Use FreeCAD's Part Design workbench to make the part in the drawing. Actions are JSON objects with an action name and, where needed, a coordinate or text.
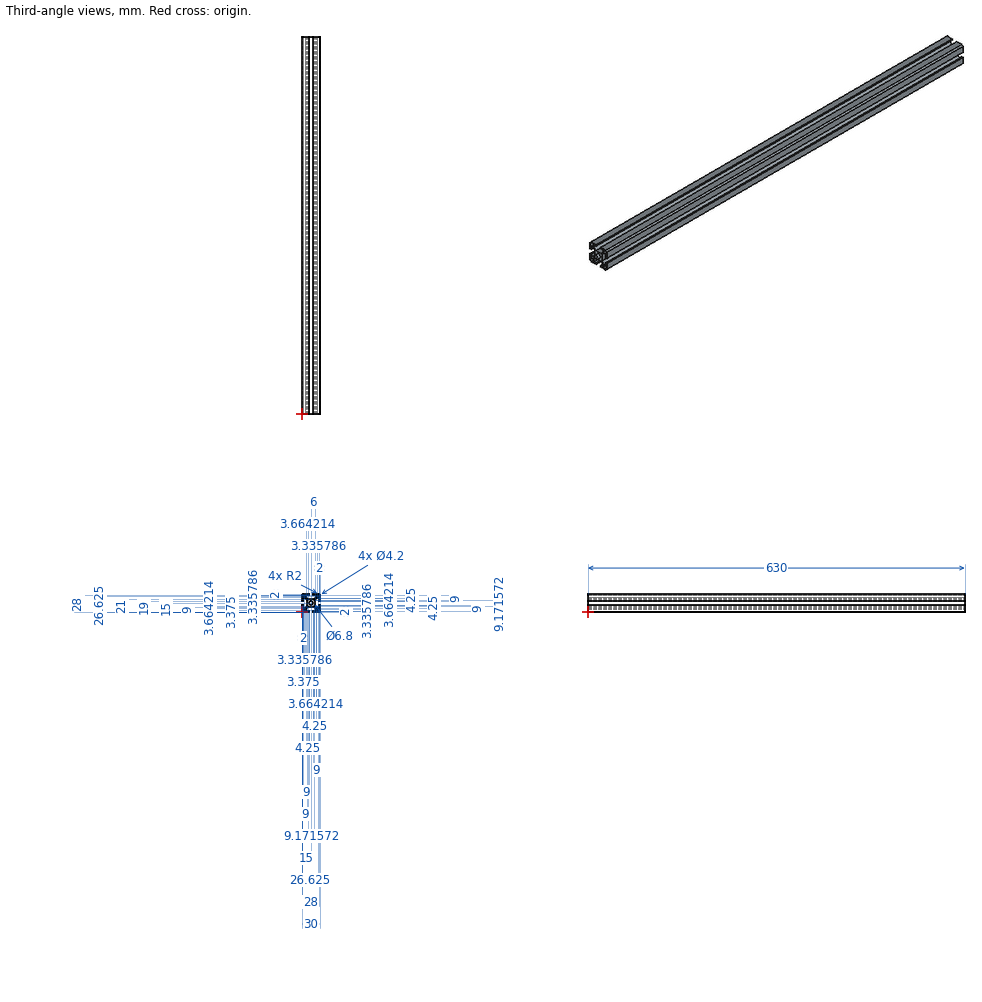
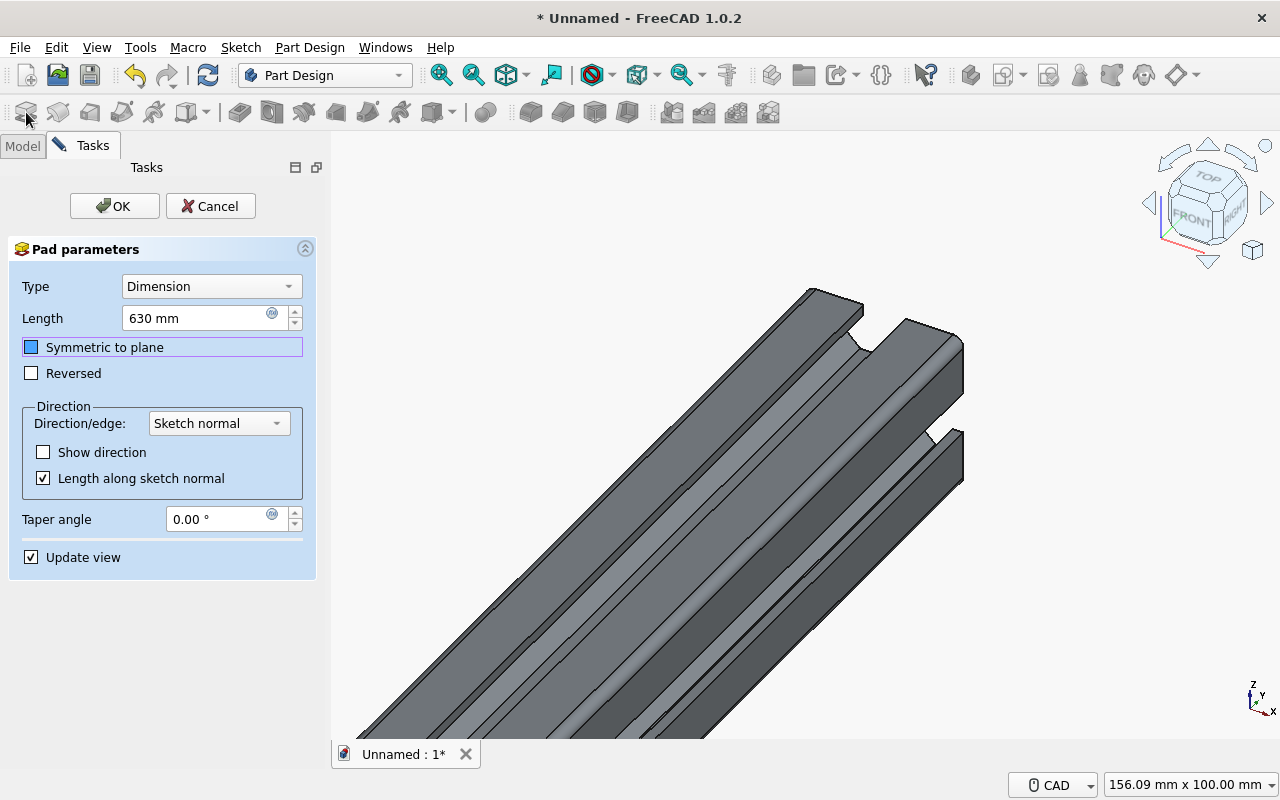
{"action": "left_click", "coordinate": [30, 373]}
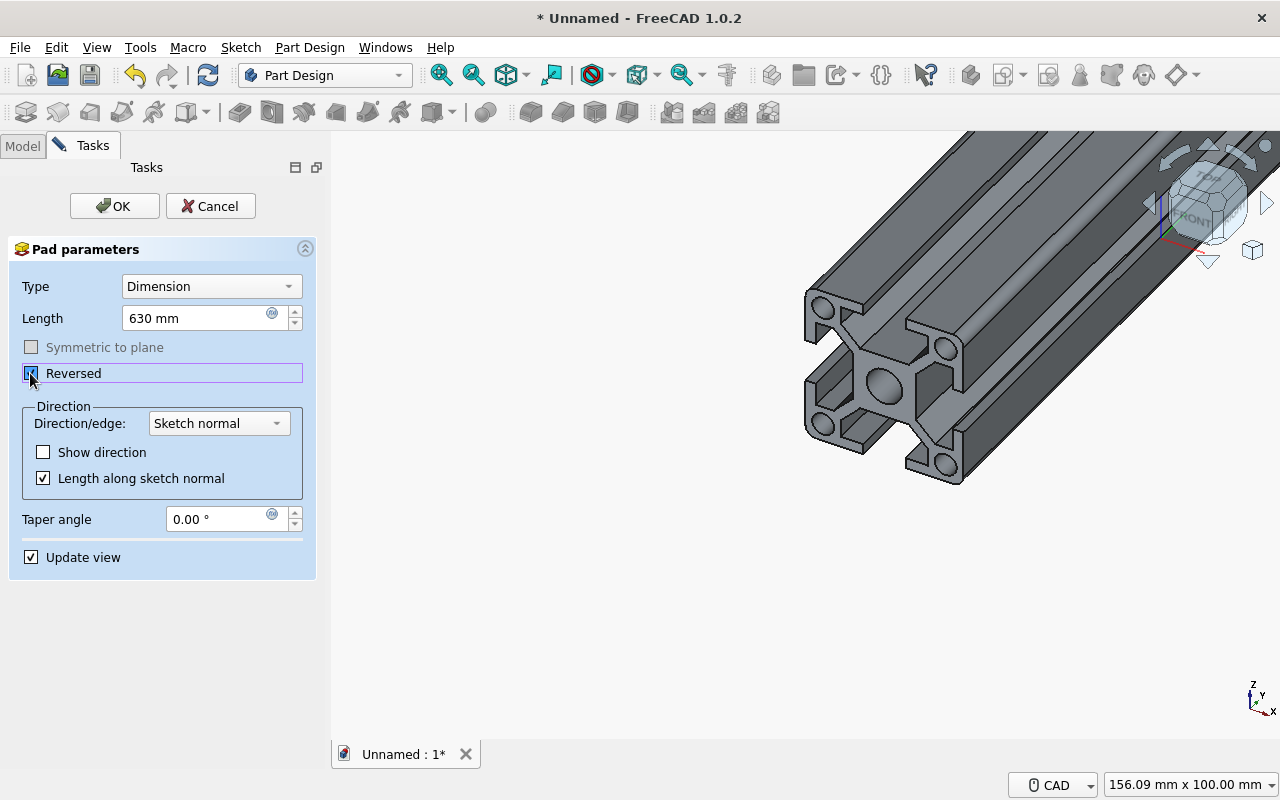
{"action": "left_click", "coordinate": [115, 206]}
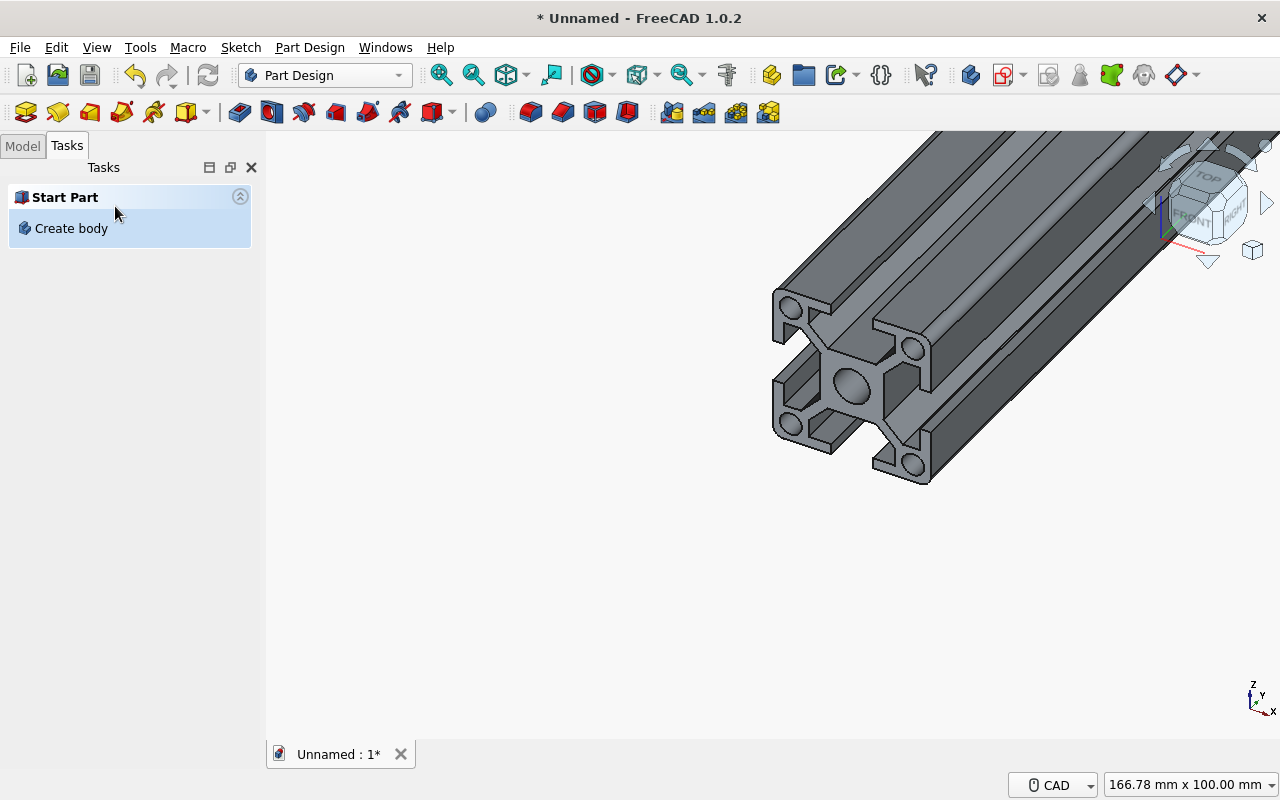
{"action": "key", "text": "0"}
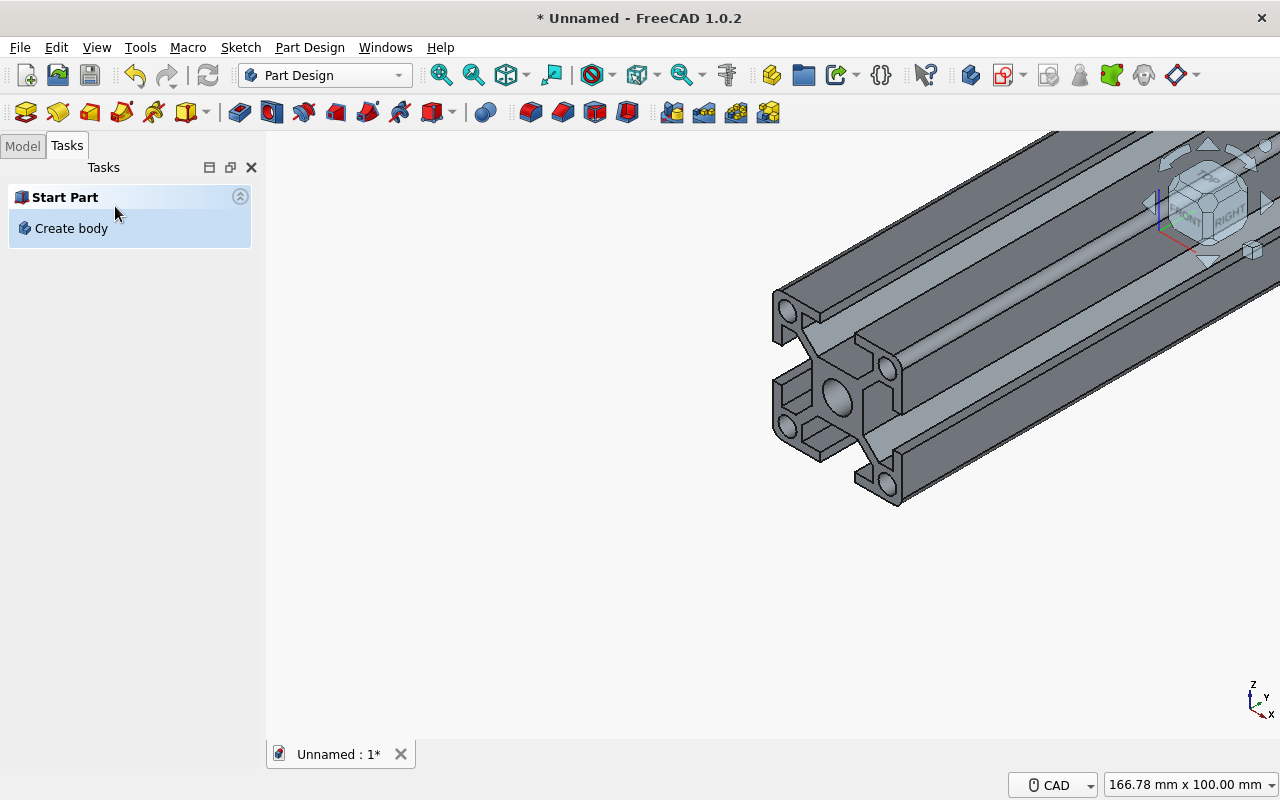
{"action": "left_click", "coordinate": [442, 76]}